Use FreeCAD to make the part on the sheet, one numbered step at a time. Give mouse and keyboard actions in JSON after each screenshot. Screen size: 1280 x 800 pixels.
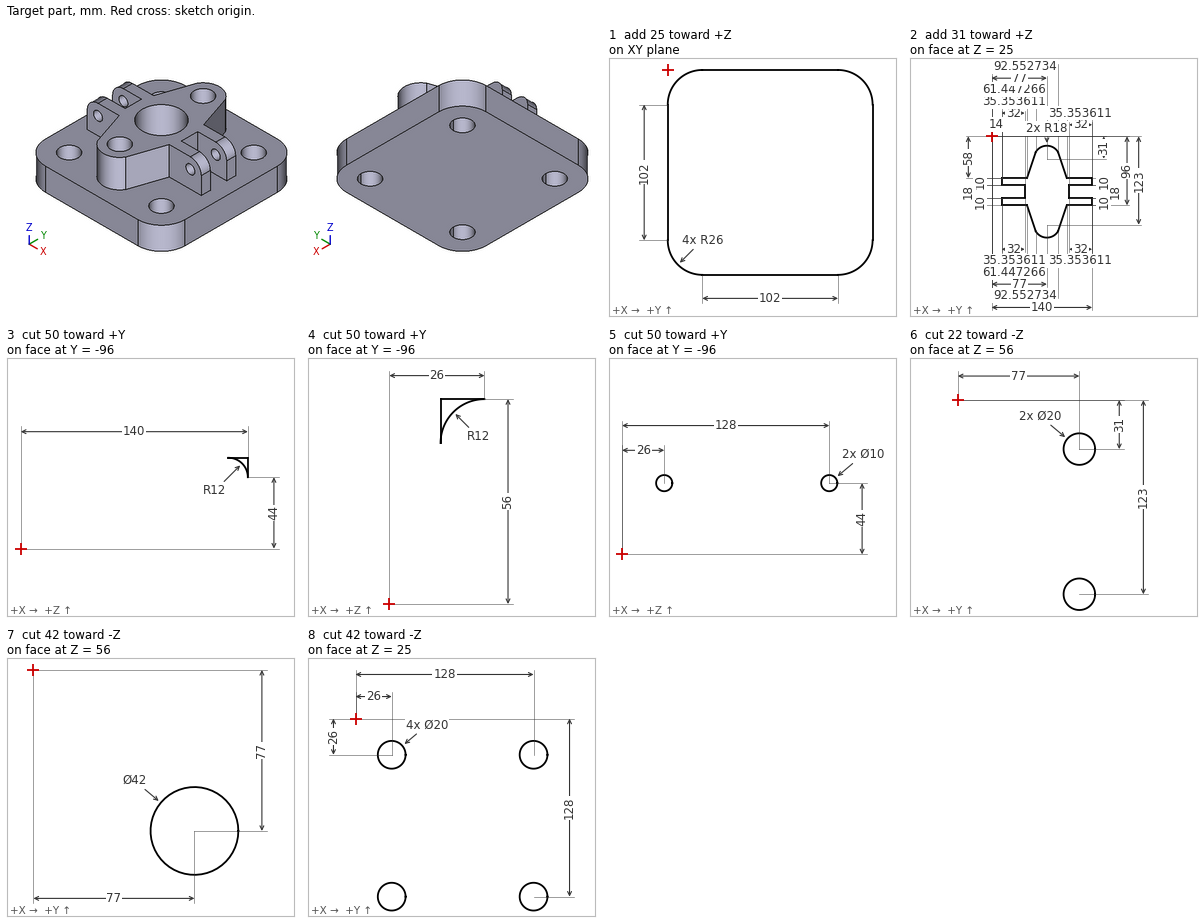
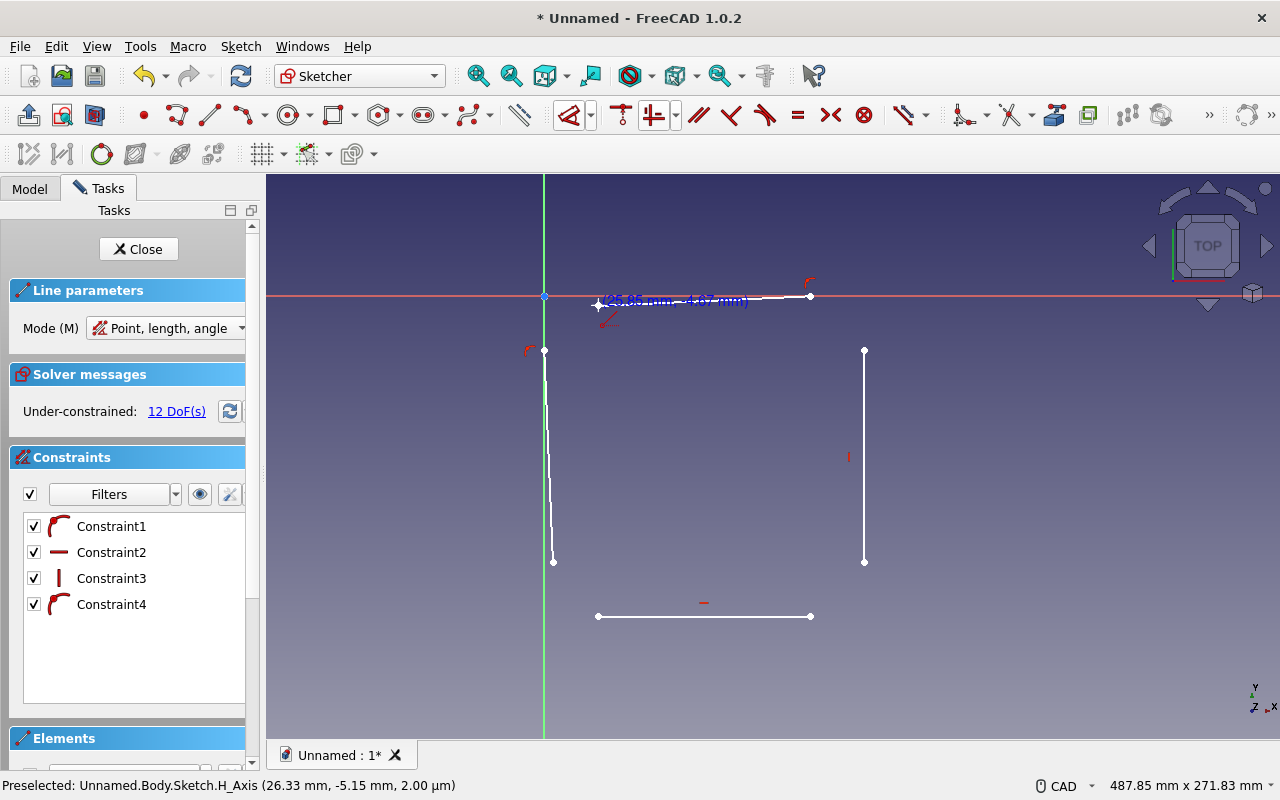
{"action": "left_click", "coordinate": [242, 116]}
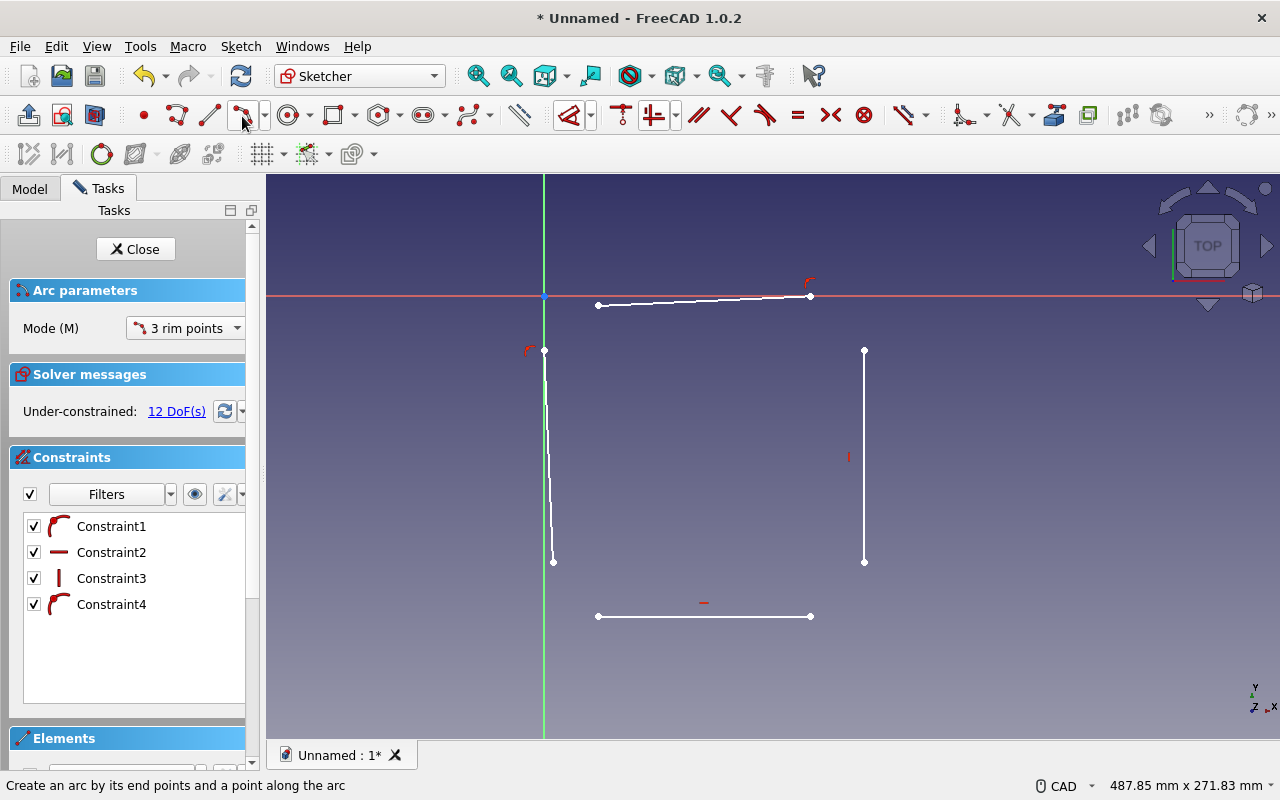
{"action": "left_click", "coordinate": [553, 563]}
{"action": "left_click", "coordinate": [598, 617]}
{"action": "left_click", "coordinate": [560, 601]}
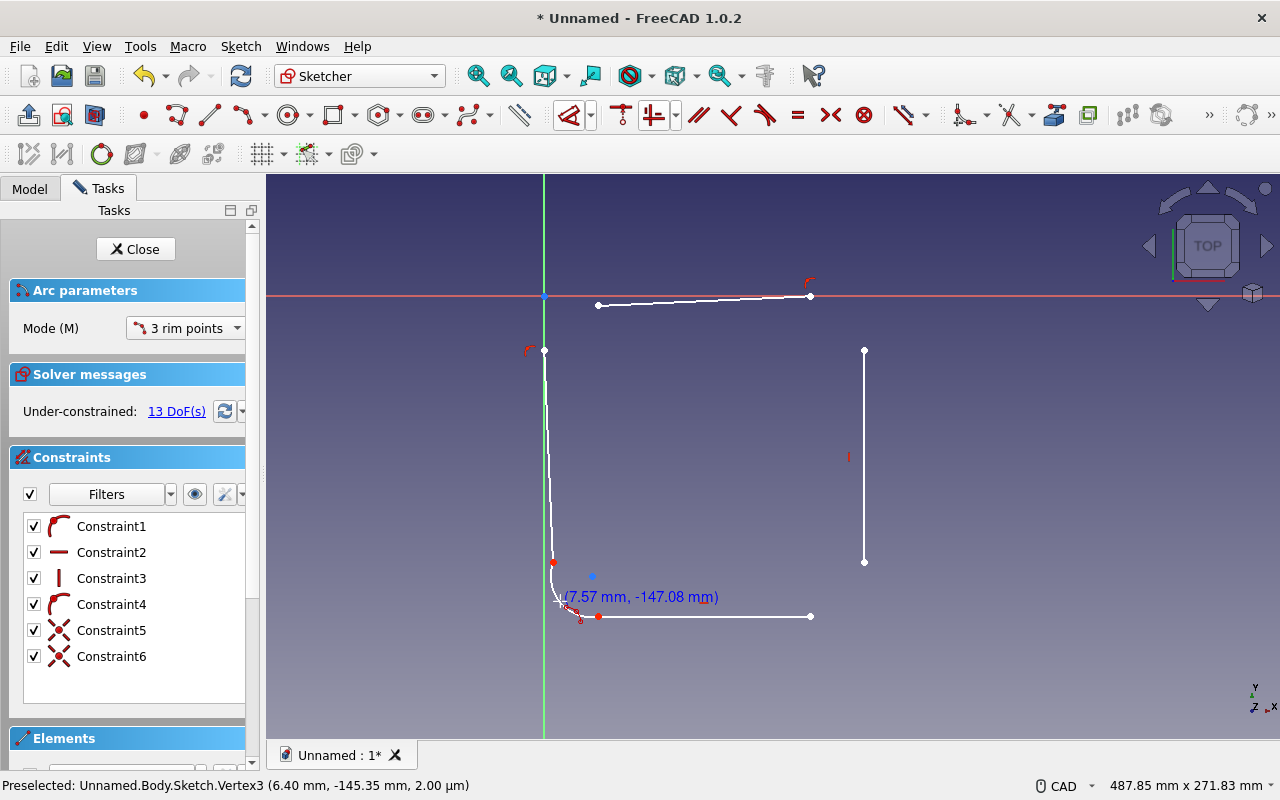
{"action": "left_click", "coordinate": [810, 617]}
{"action": "left_click", "coordinate": [864, 563]}
{"action": "left_click", "coordinate": [849, 601]}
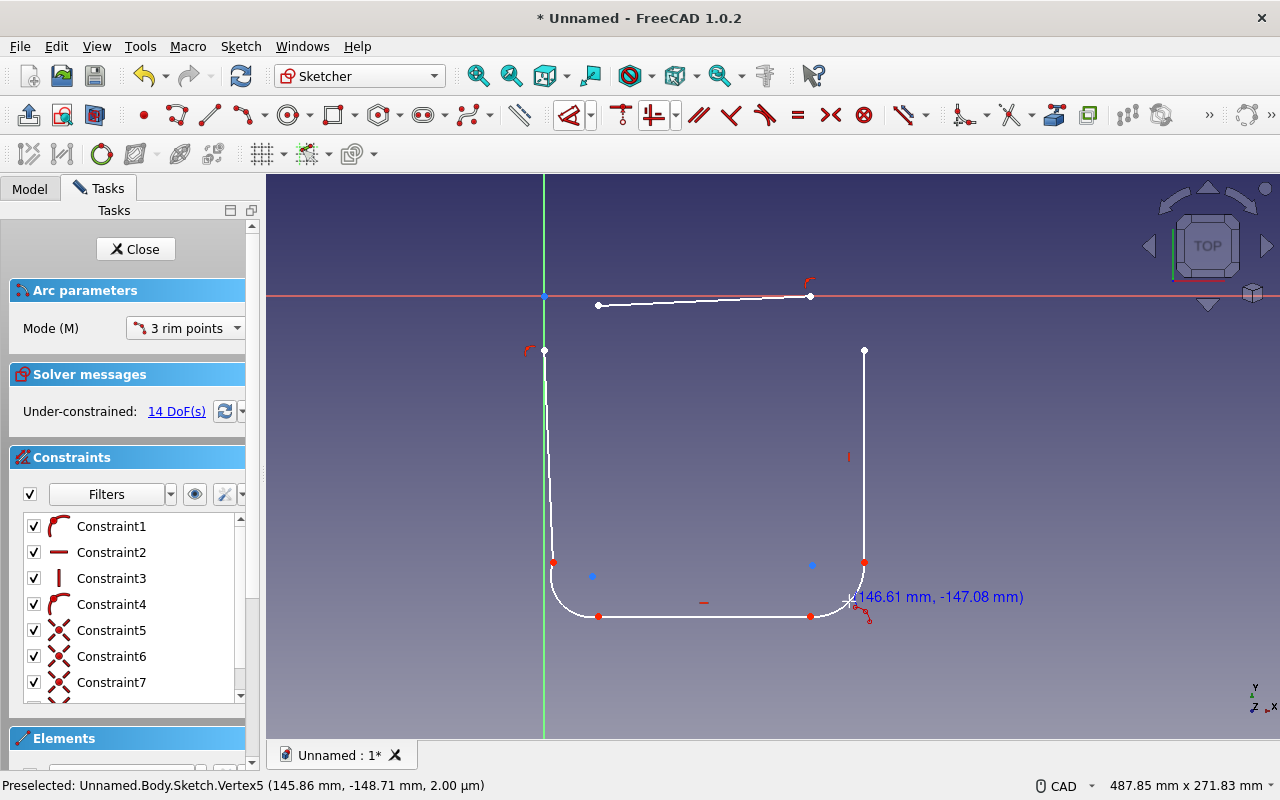
{"action": "left_click", "coordinate": [864, 351]}
{"action": "left_click", "coordinate": [810, 296]}
{"action": "left_click", "coordinate": [849, 312]}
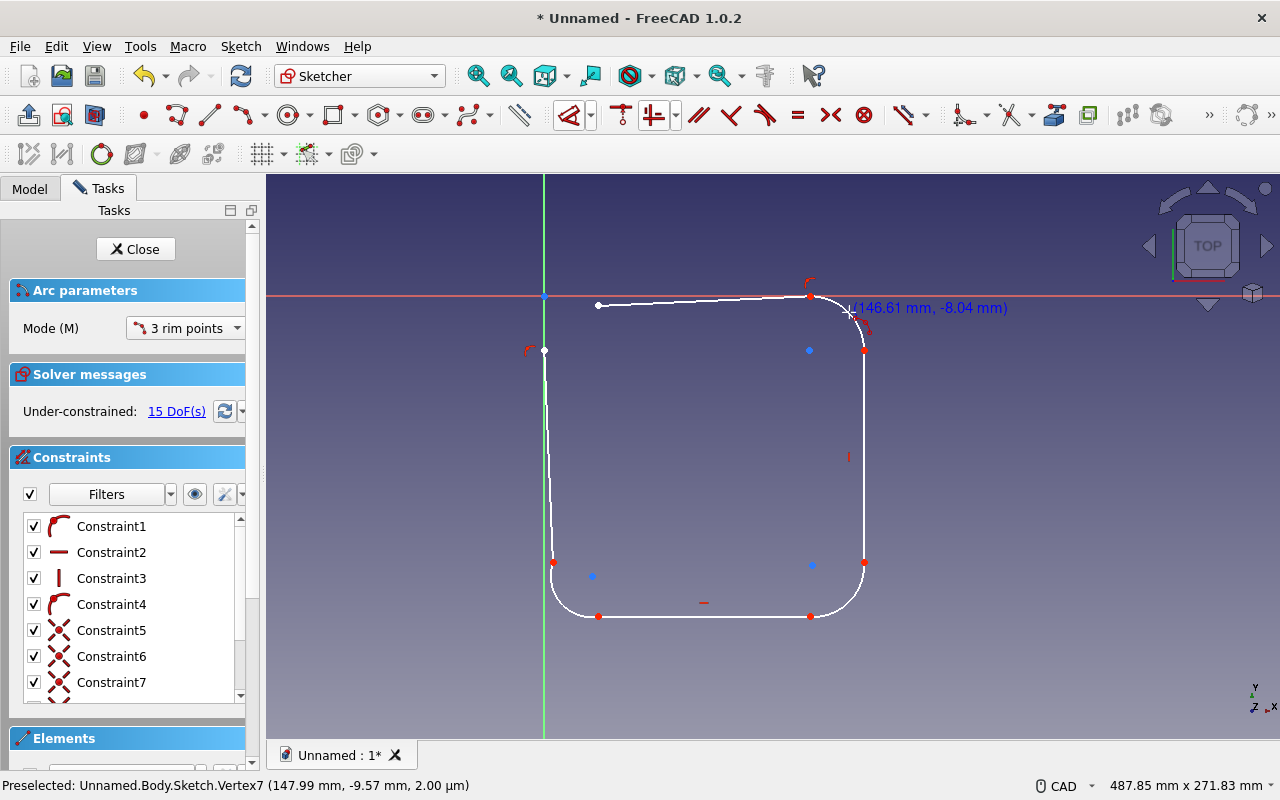
{"action": "left_click", "coordinate": [598, 306]}
{"action": "left_click", "coordinate": [544, 351]}
{"action": "left_click", "coordinate": [560, 312]}
{"action": "key", "text": "Escape"}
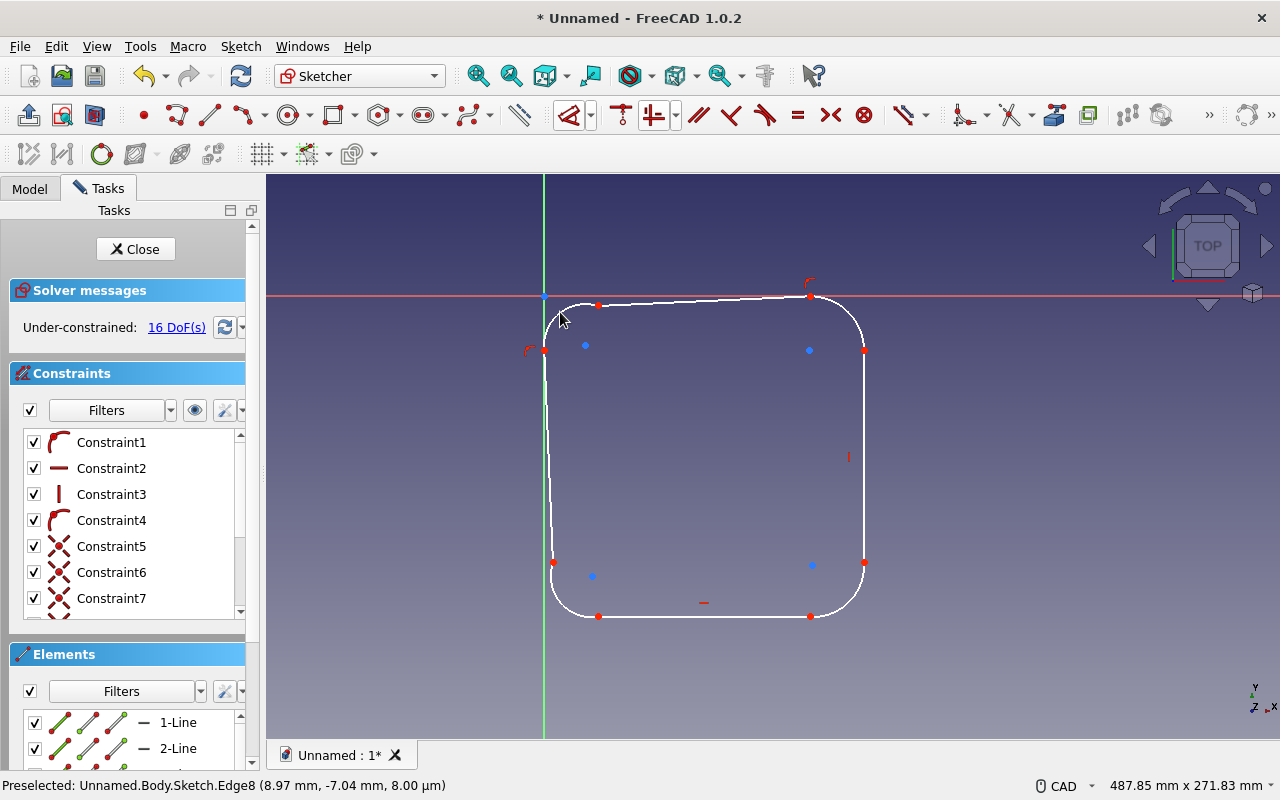
{"action": "left_click", "coordinate": [547, 415]}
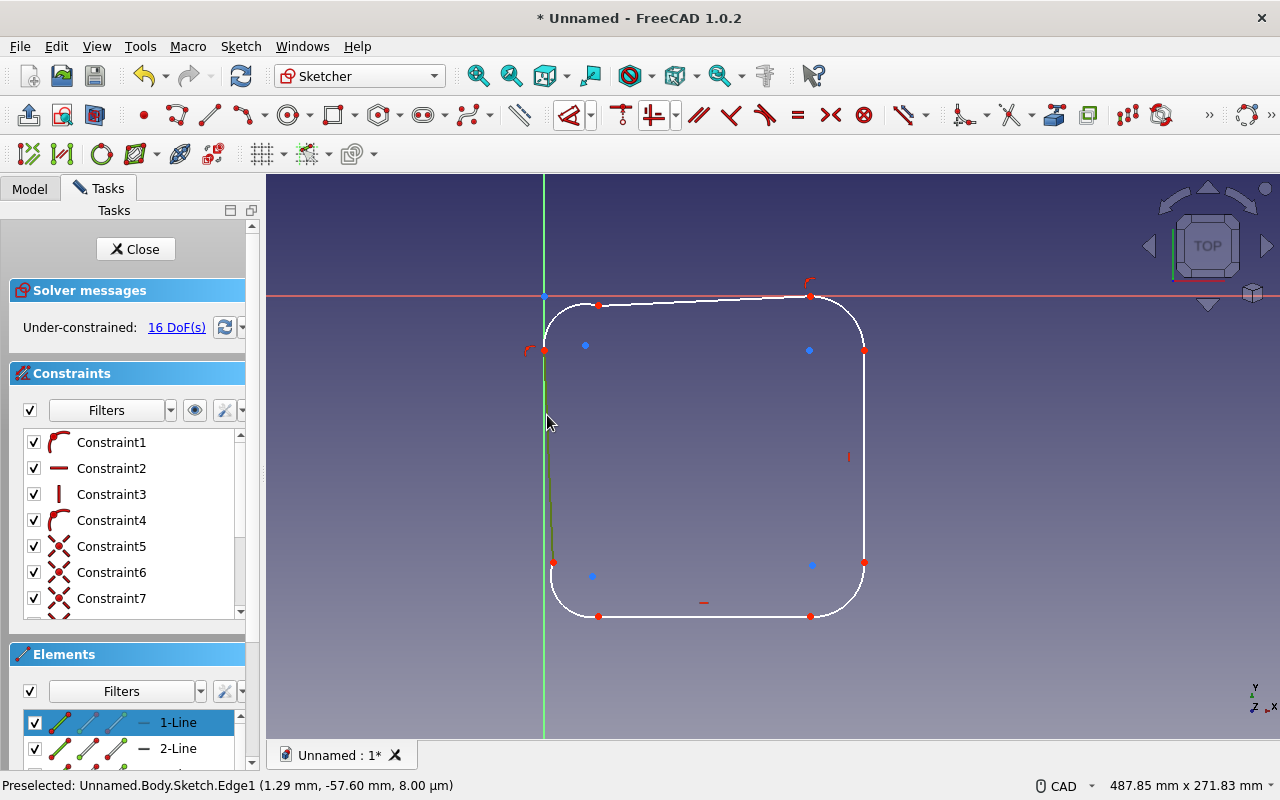
{"action": "left_click", "coordinate": [574, 613]}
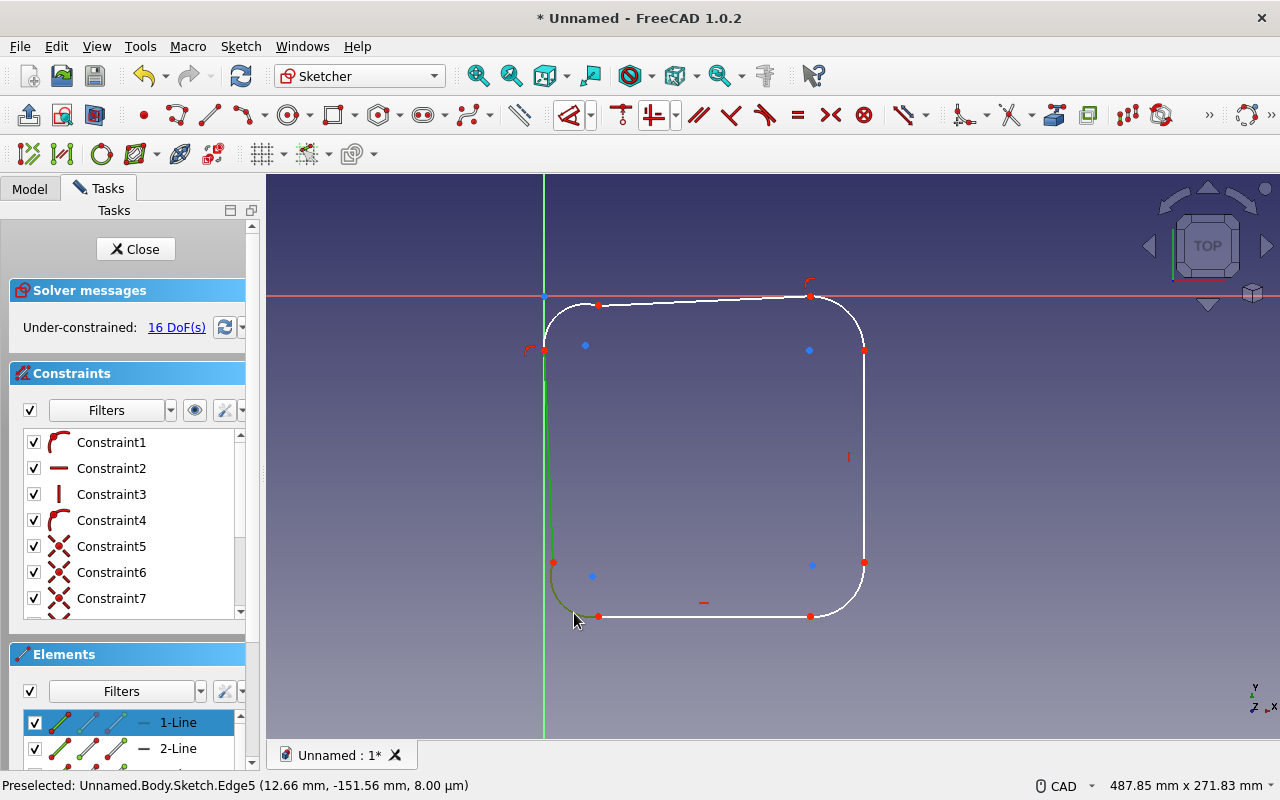
{"action": "left_click", "coordinate": [765, 116]}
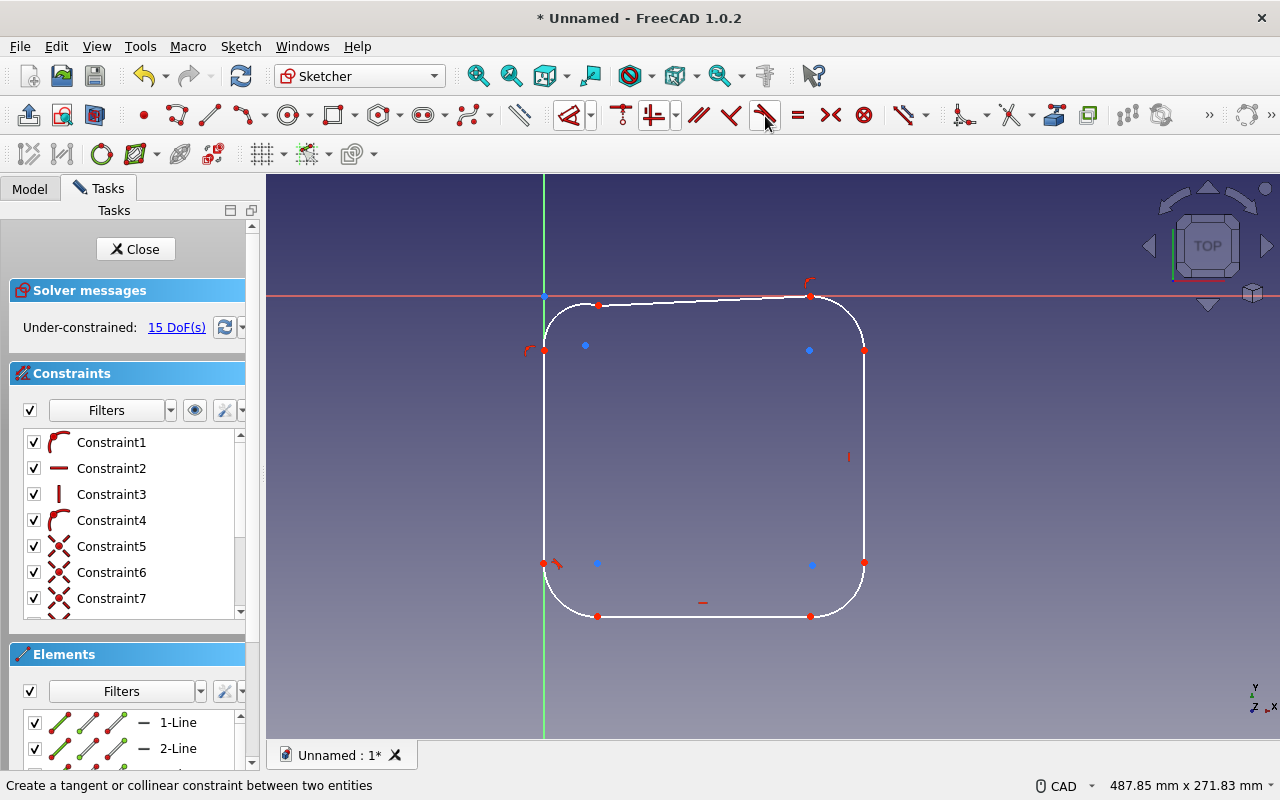
{"action": "left_click", "coordinate": [544, 415]}